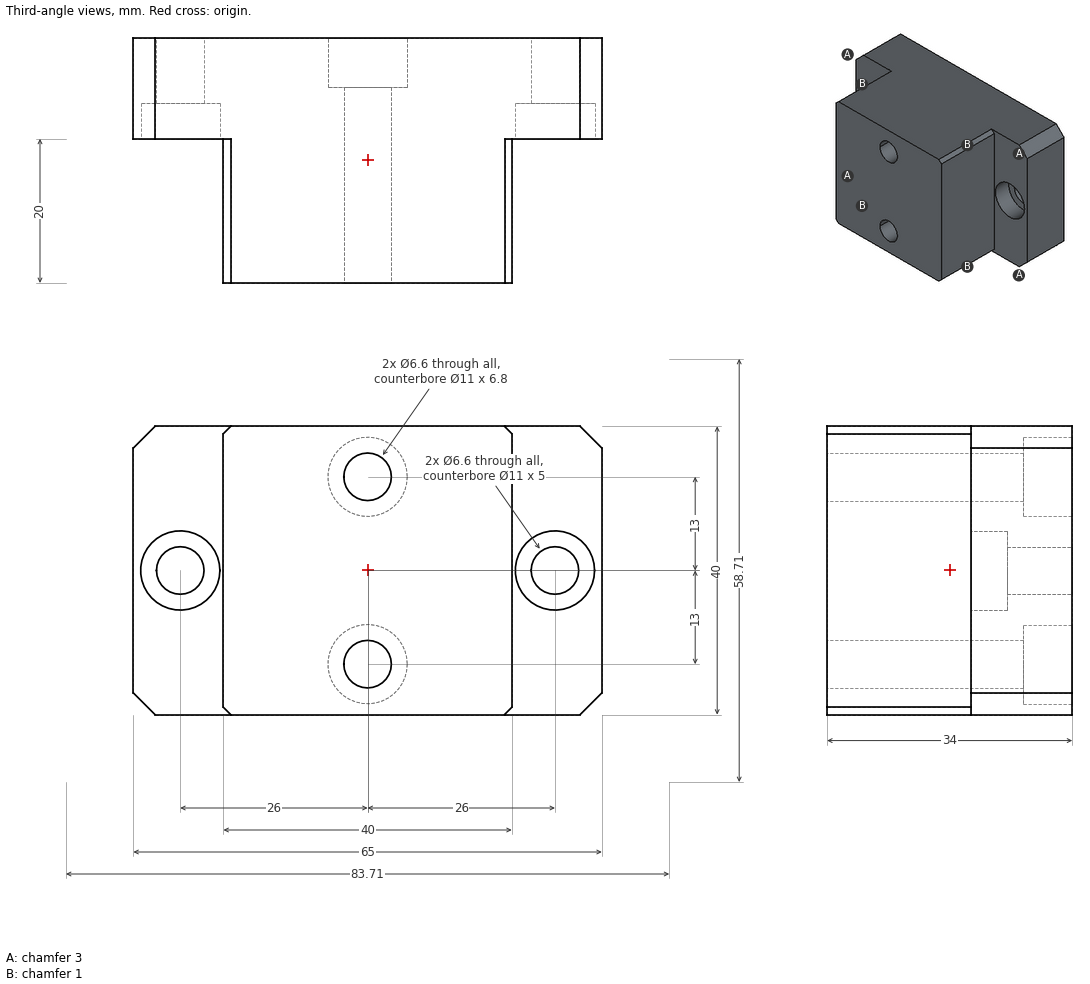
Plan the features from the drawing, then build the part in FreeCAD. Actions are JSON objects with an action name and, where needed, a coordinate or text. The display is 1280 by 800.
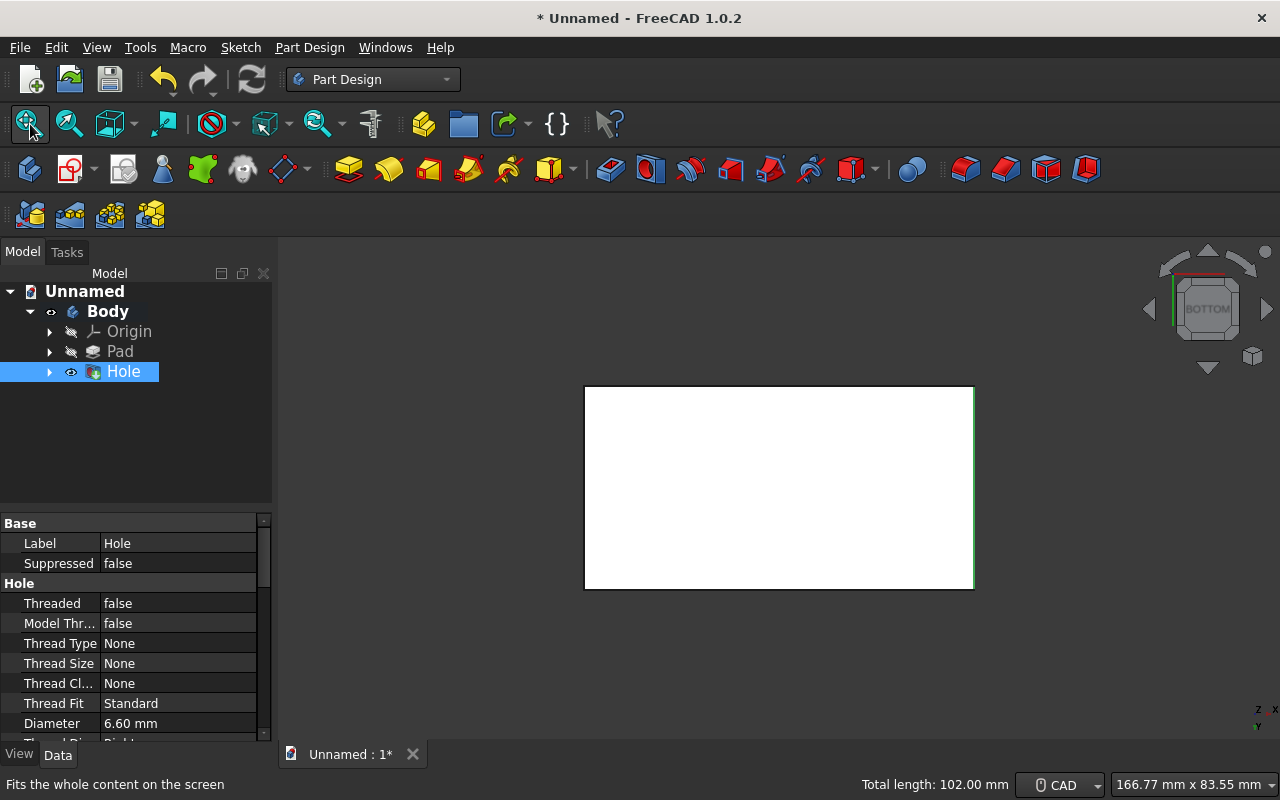
{"action": "left_click", "coordinate": [584, 487], "text": "ctrl"}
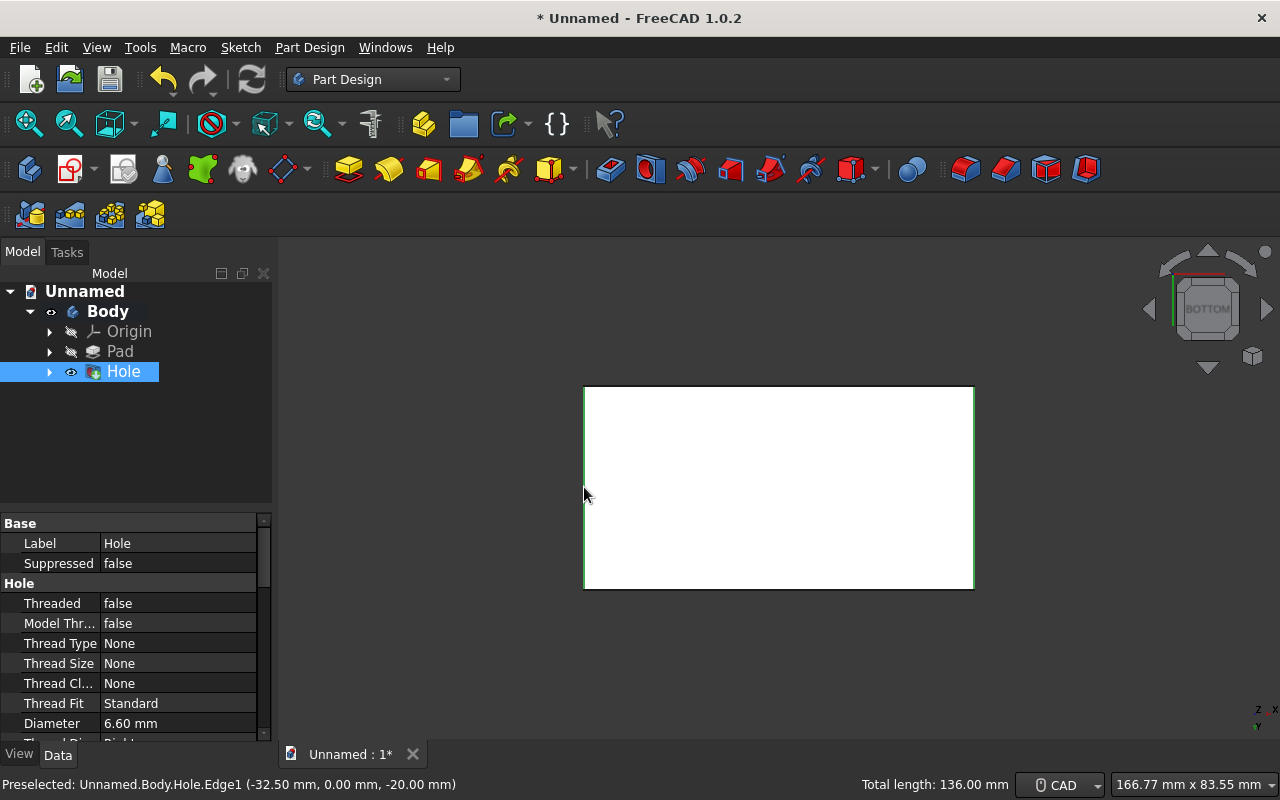
{"action": "left_click", "coordinate": [1006, 170]}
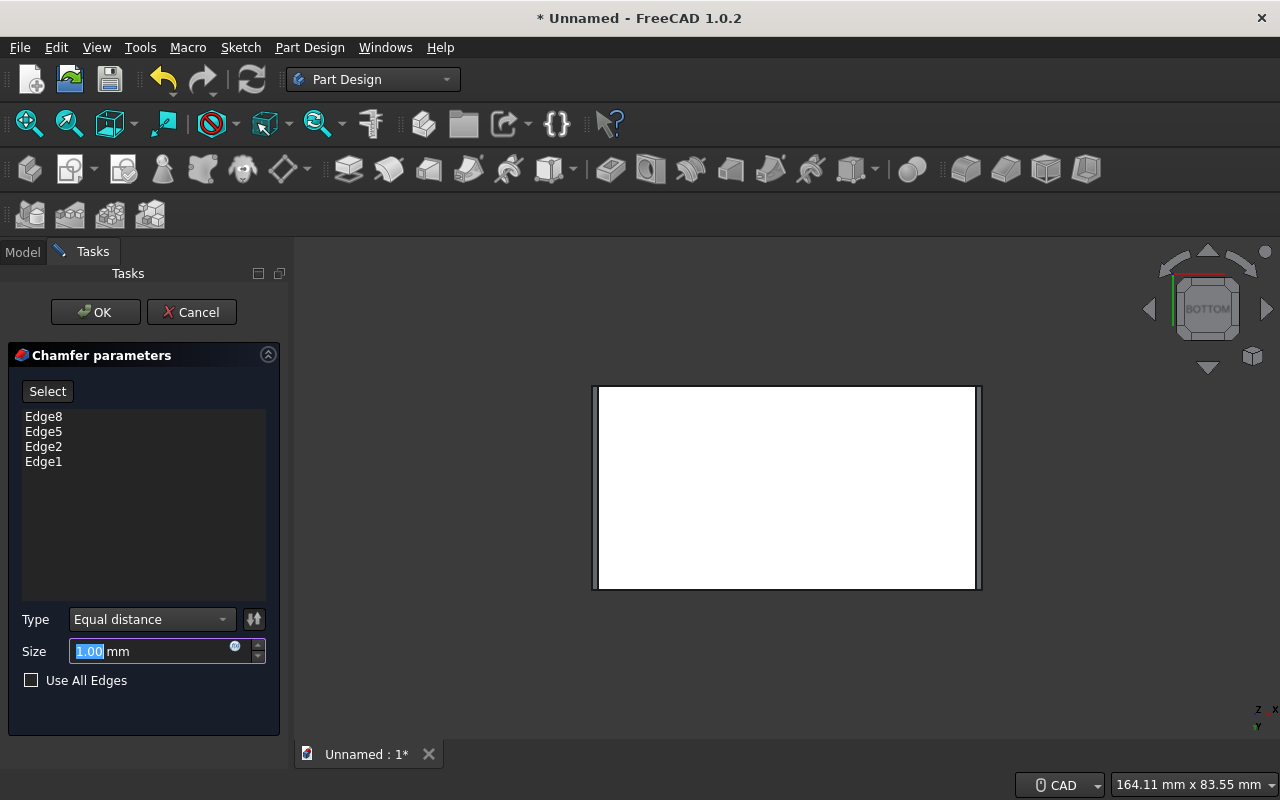
{"action": "type", "text": "3"}
{"action": "key", "text": "Tab"}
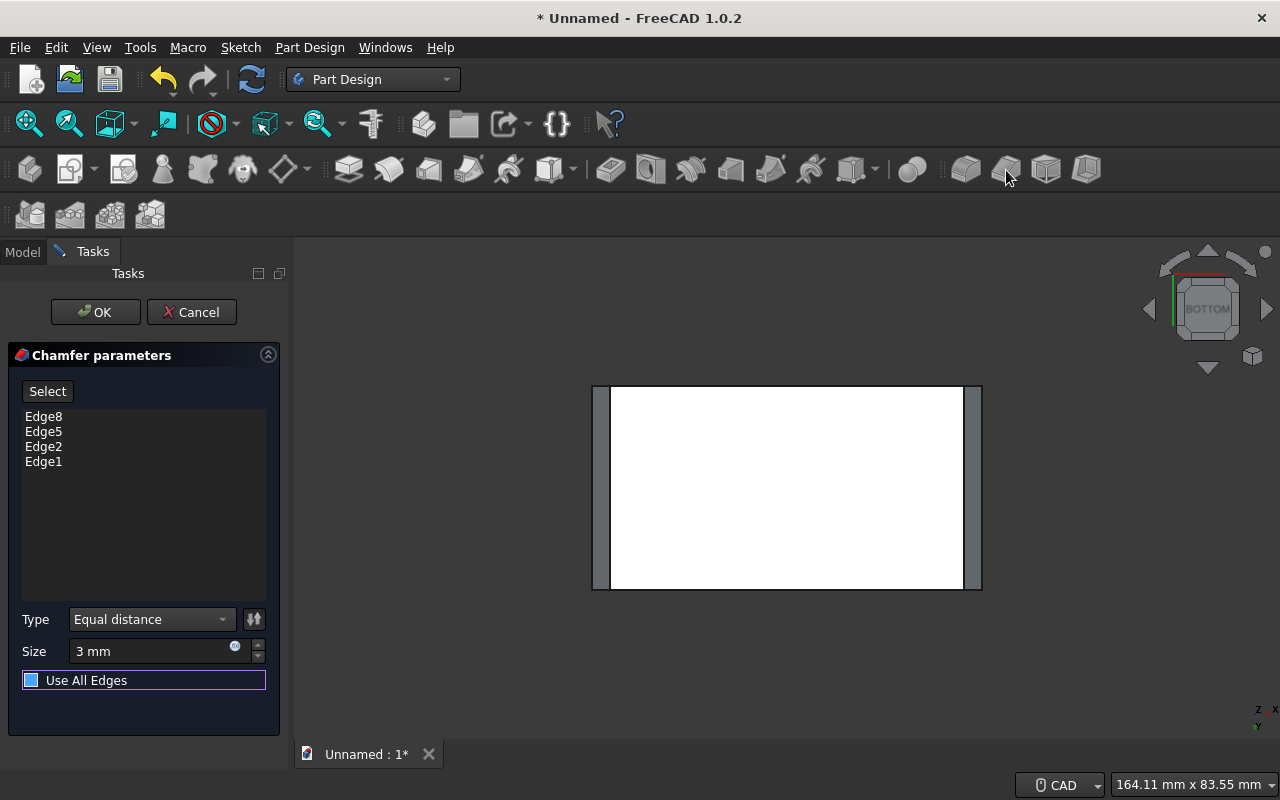
{"action": "left_click", "coordinate": [96, 312]}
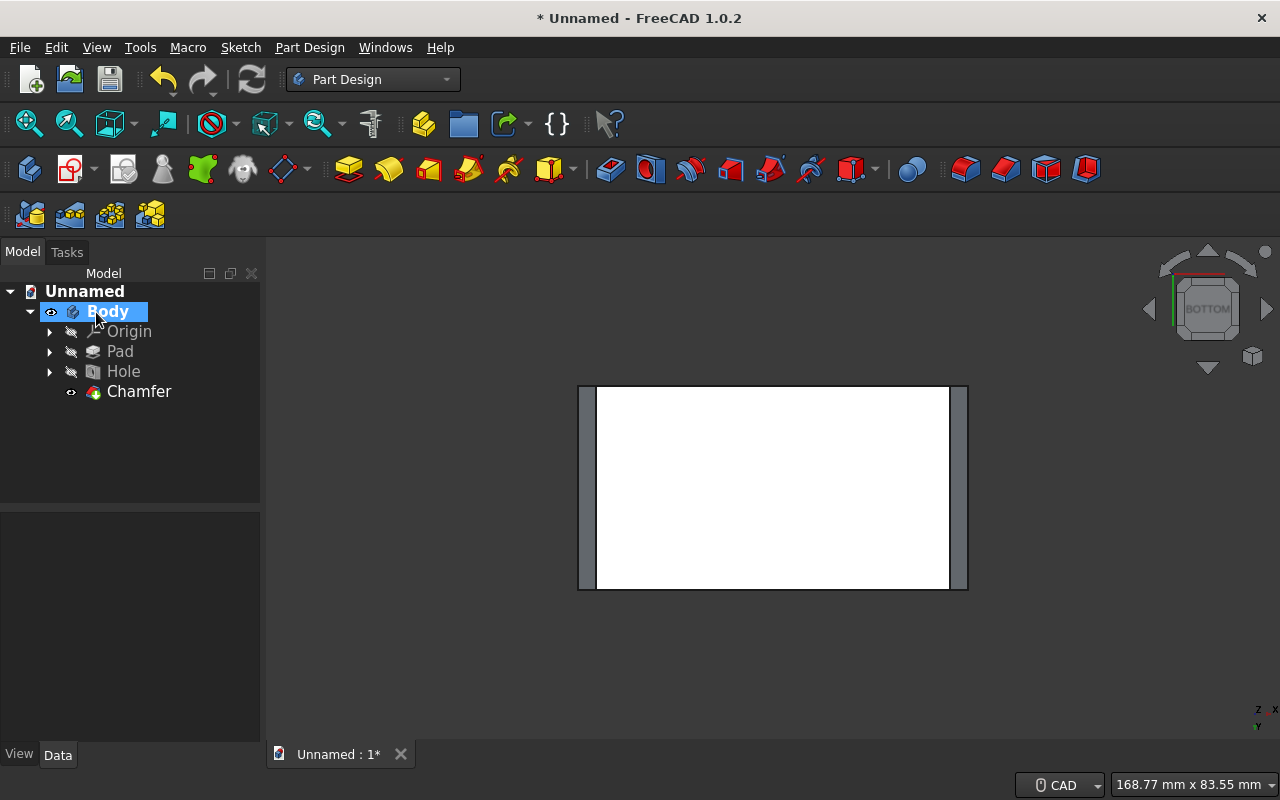
{"action": "left_click", "coordinate": [30, 124]}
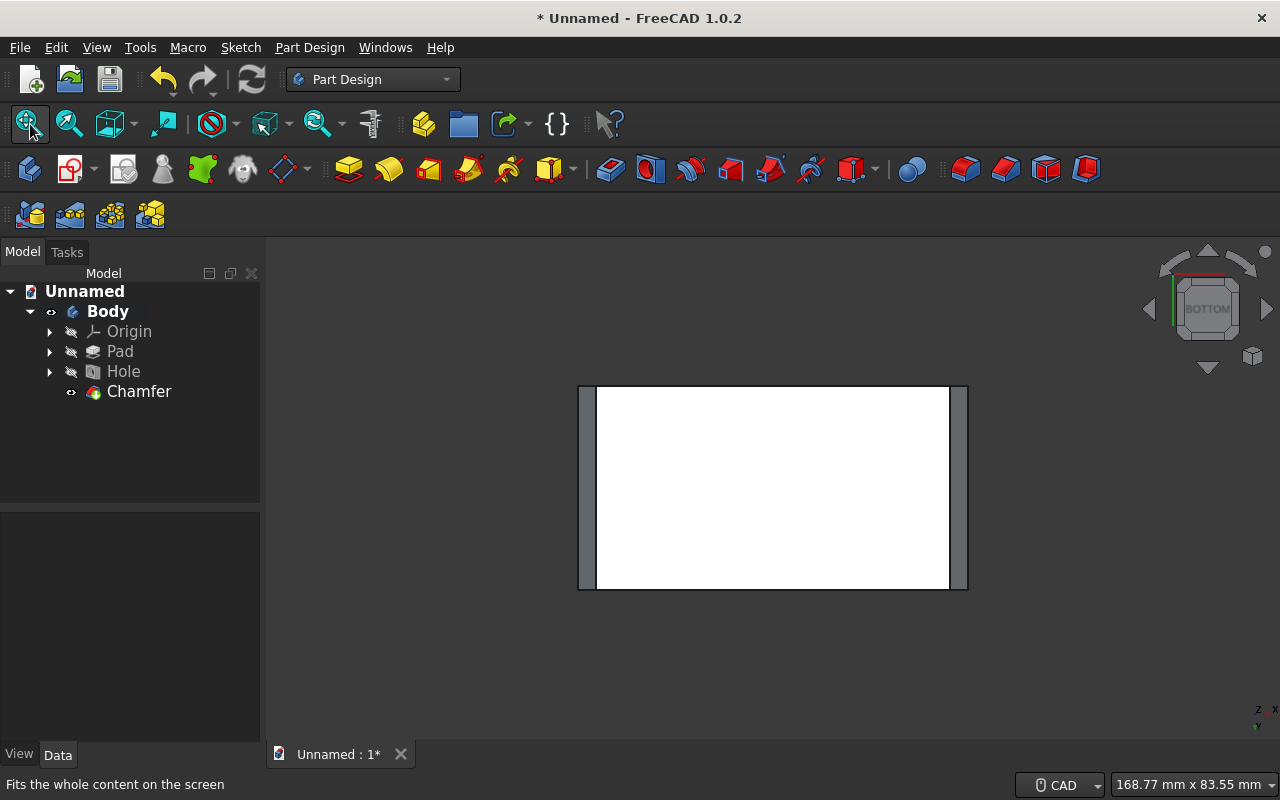
{"action": "key", "text": "0"}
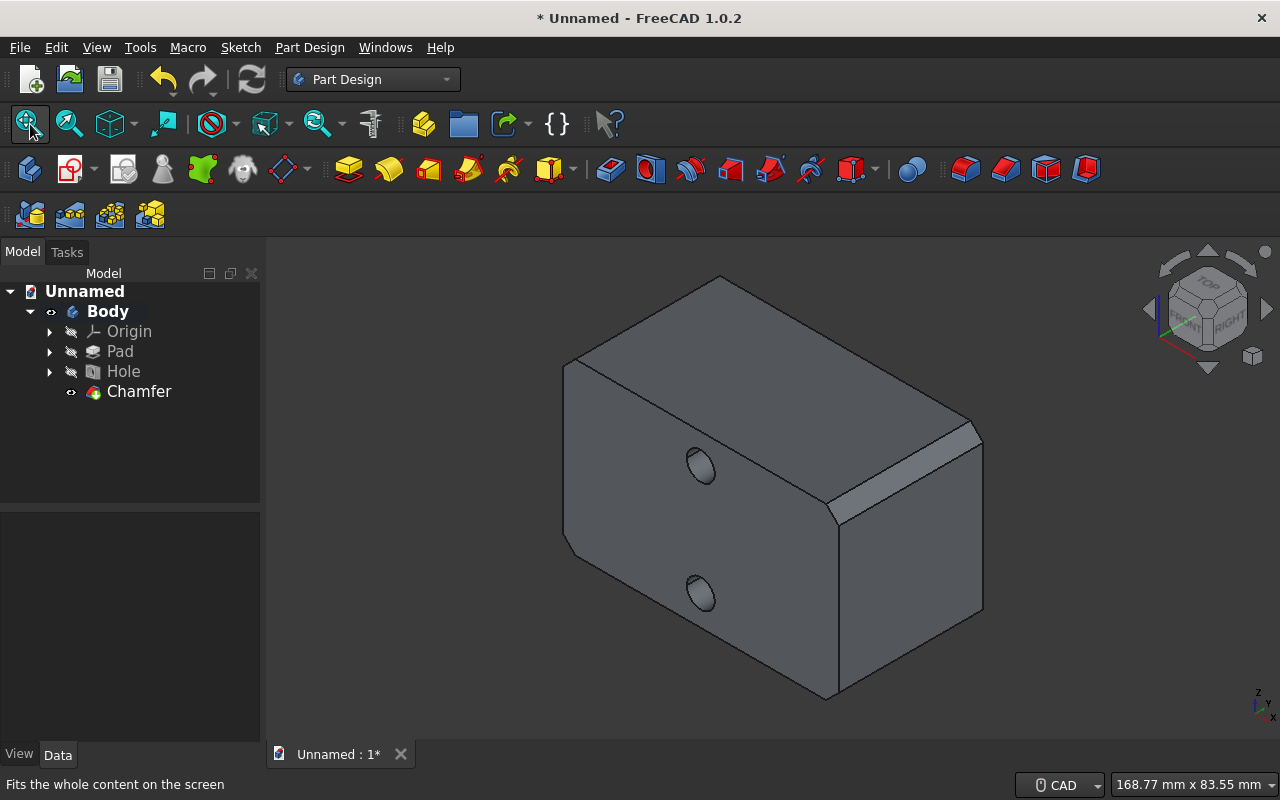
{"action": "left_click", "coordinate": [780, 546]}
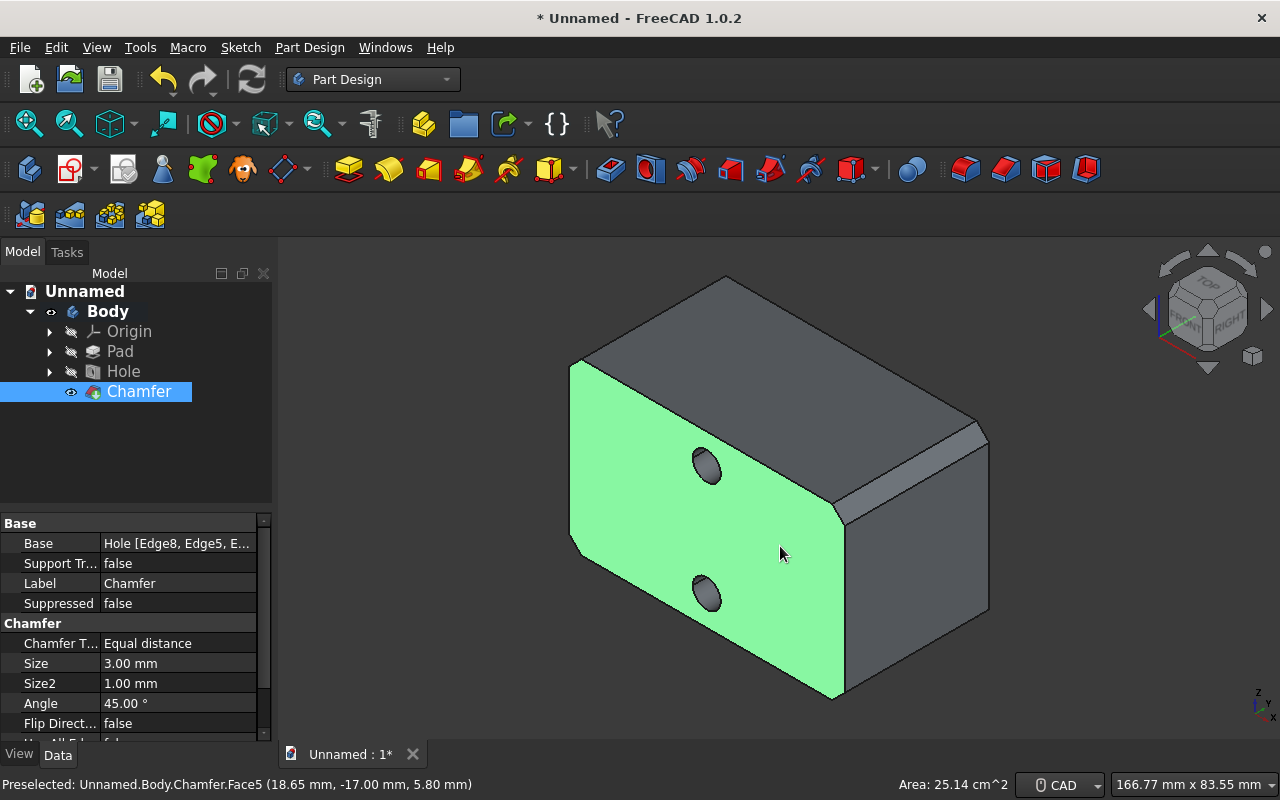
{"action": "left_click", "coordinate": [70, 170]}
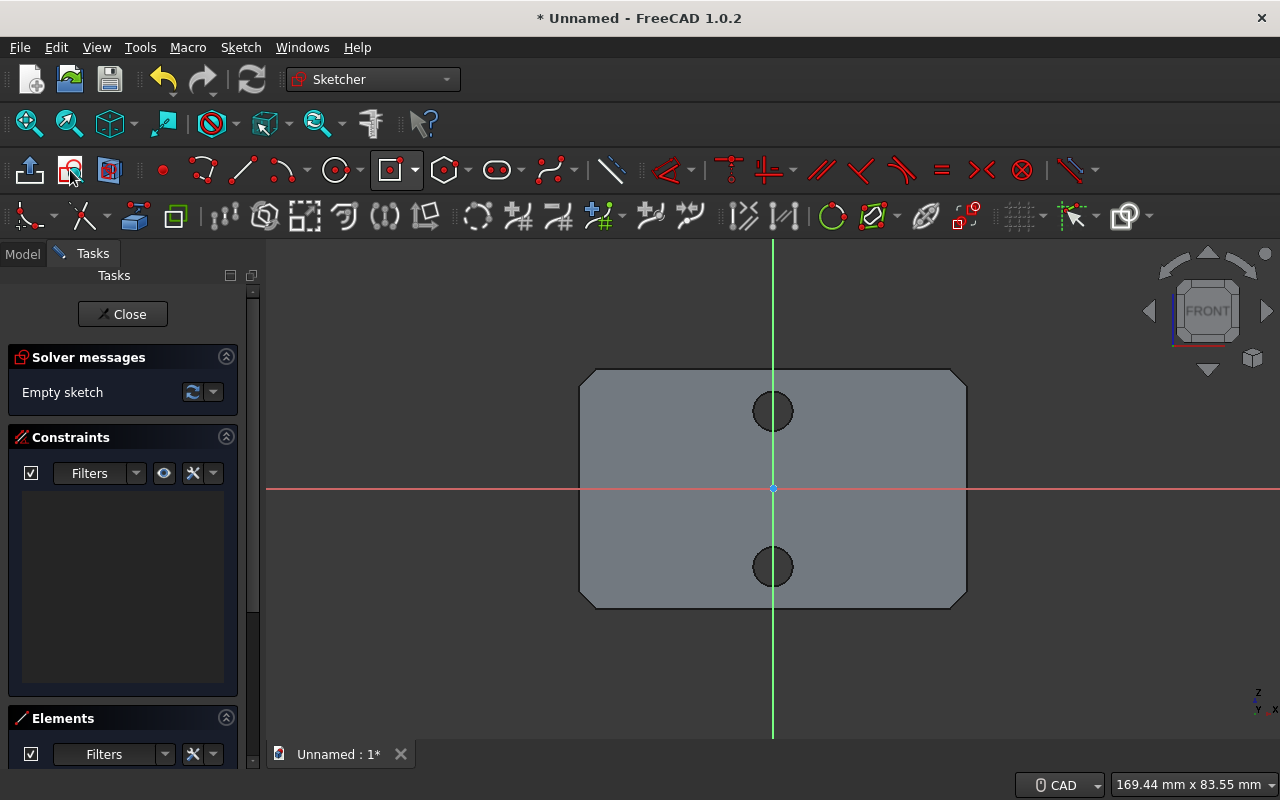
{"action": "left_click", "coordinate": [390, 170]}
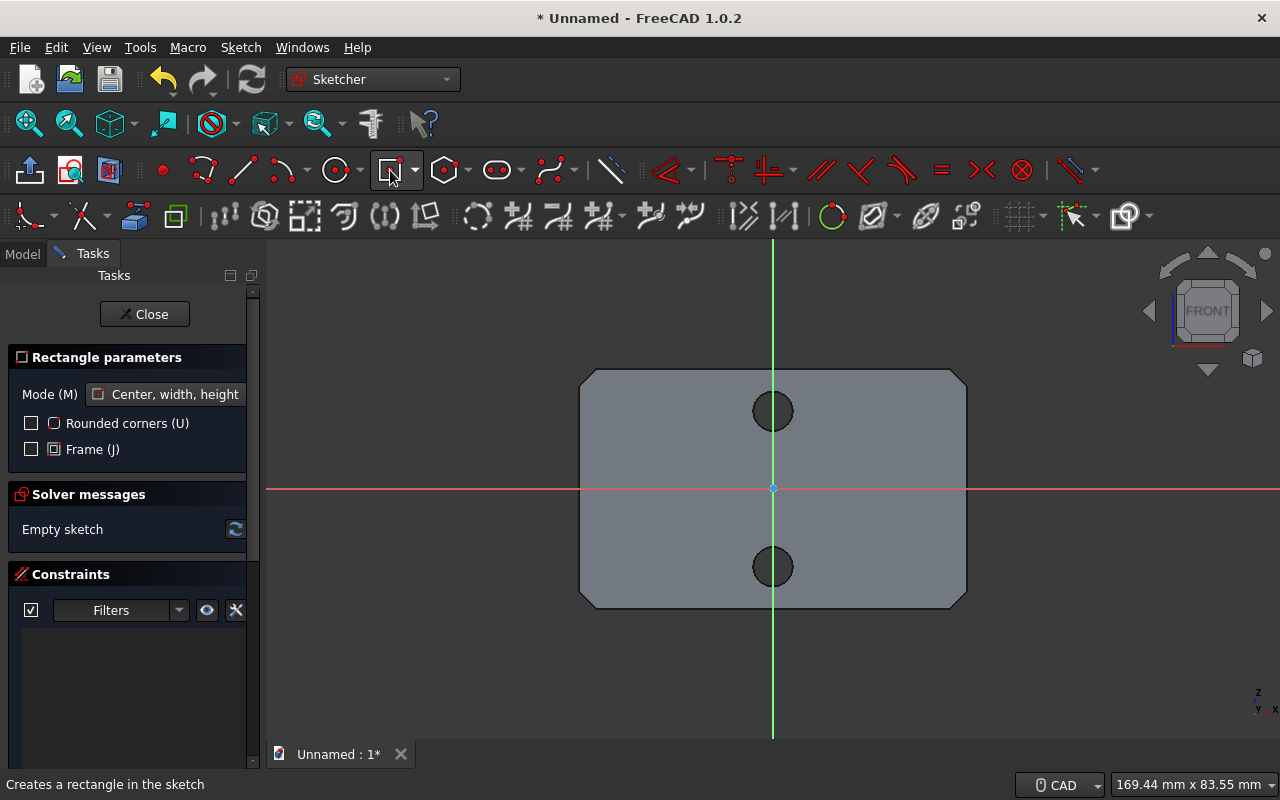
{"action": "left_click", "coordinate": [773, 489]}
{"action": "left_click", "coordinate": [1023, 313]}